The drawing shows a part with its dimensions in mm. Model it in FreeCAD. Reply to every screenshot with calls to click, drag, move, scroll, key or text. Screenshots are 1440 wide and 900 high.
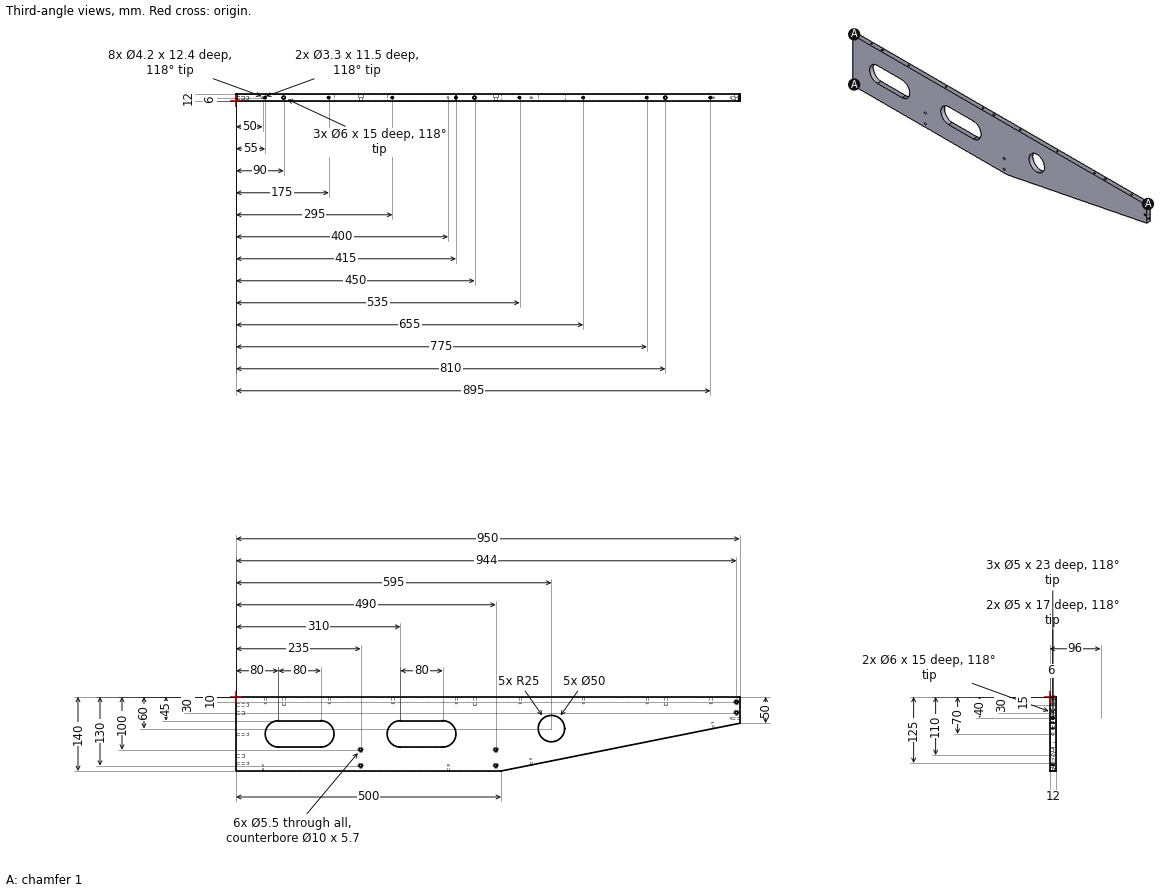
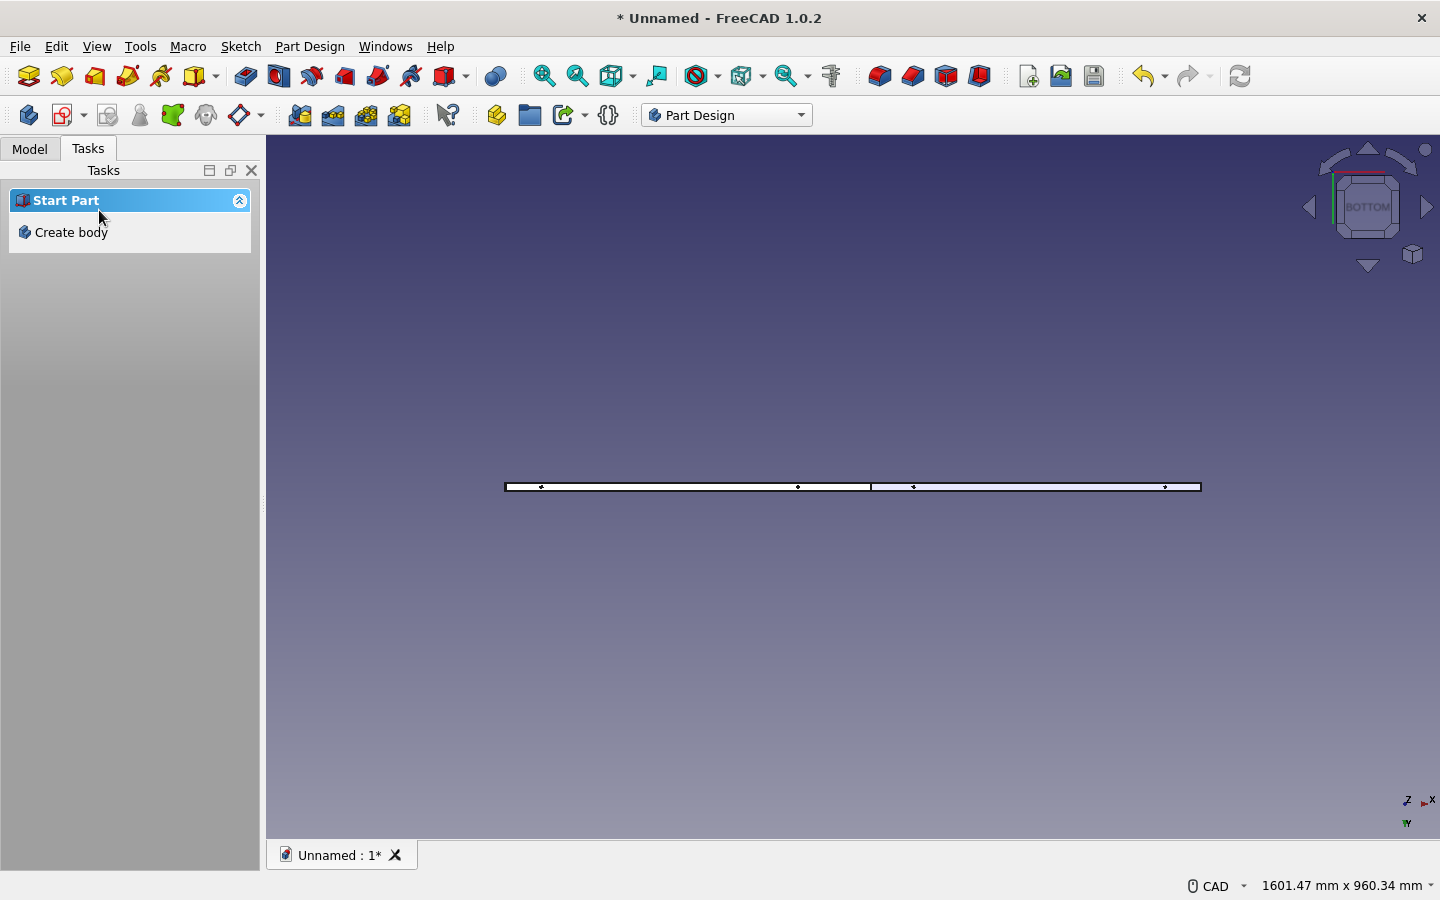
key(0)